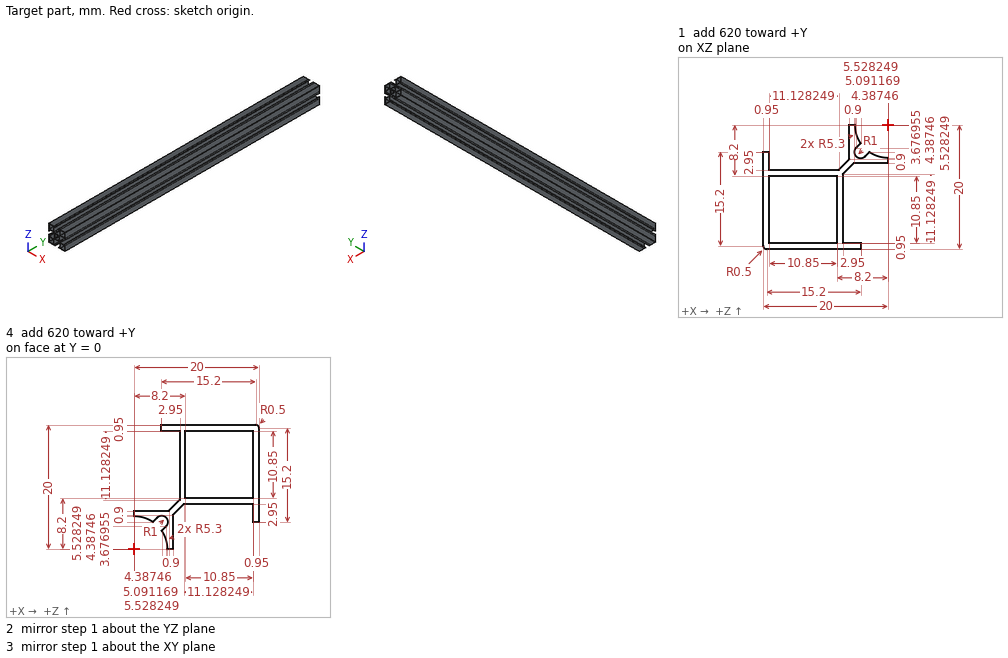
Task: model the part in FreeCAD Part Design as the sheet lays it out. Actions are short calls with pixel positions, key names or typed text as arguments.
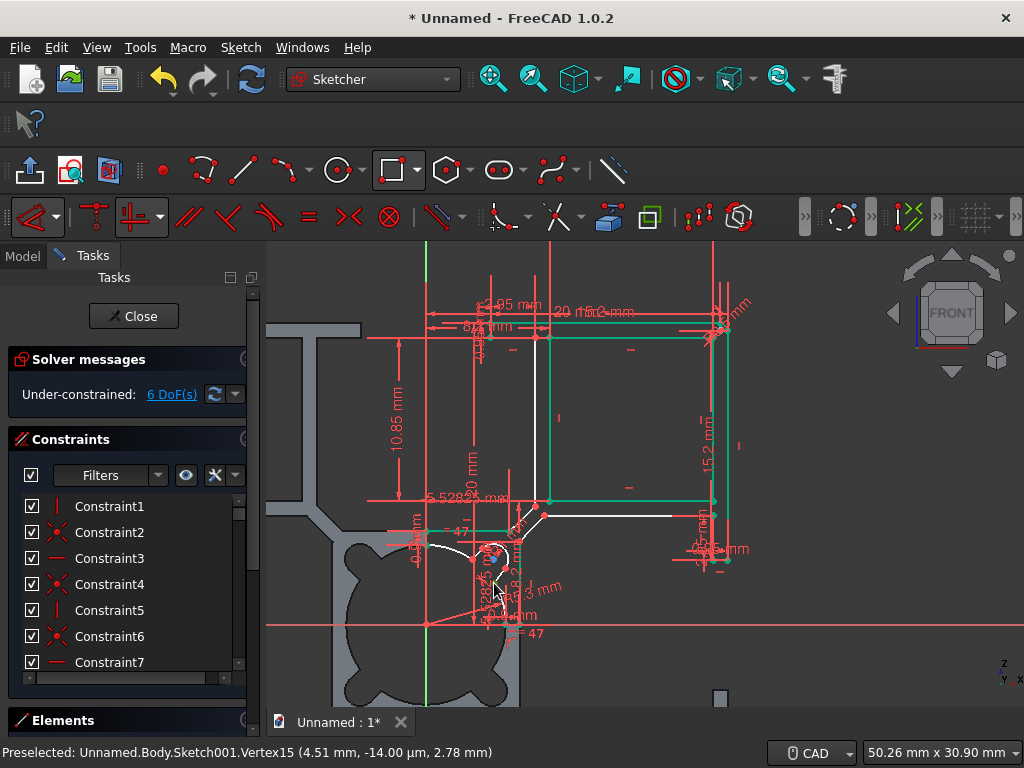
click(58, 218)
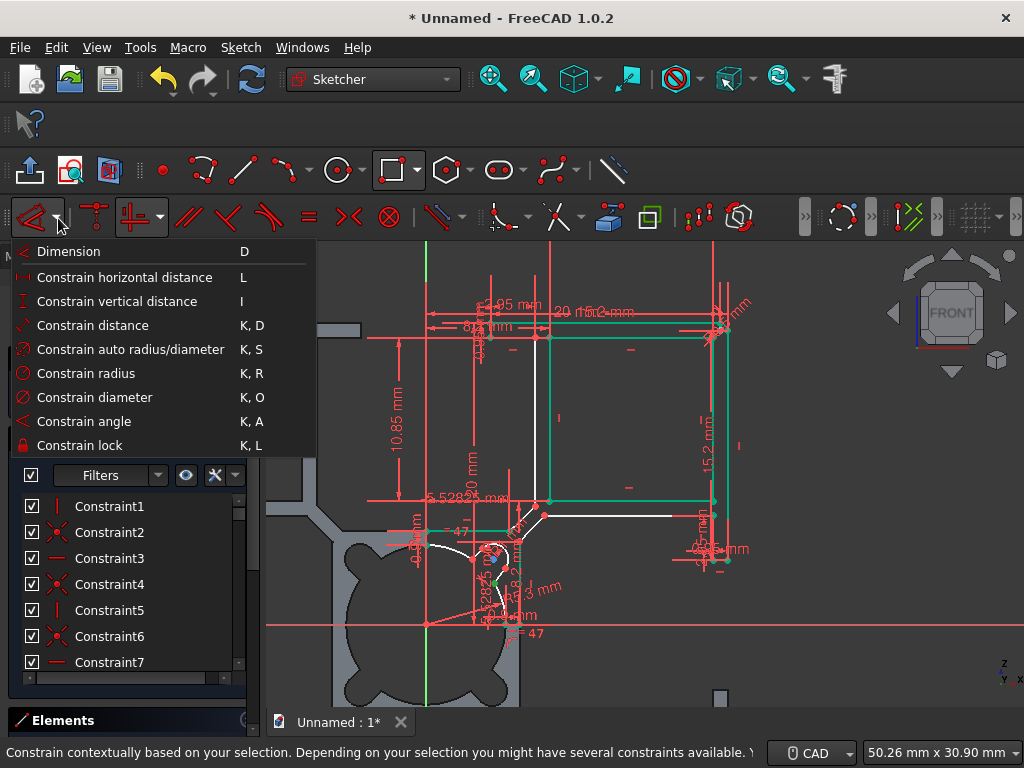
click(164, 277)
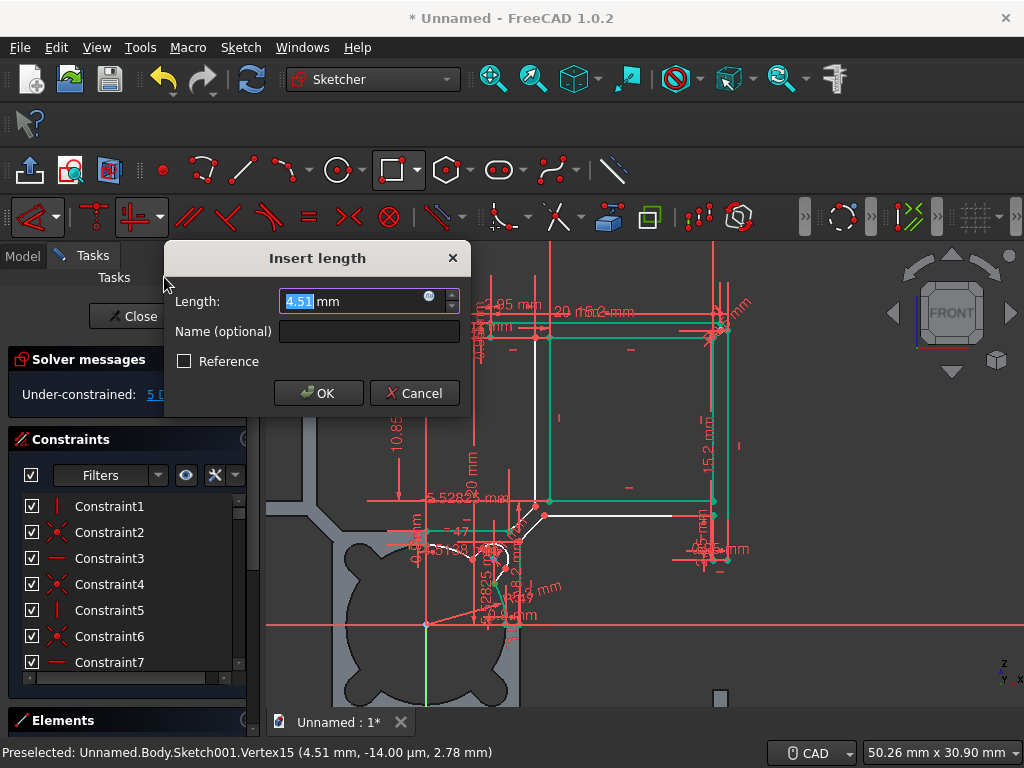
text(4.38746)
key(Return)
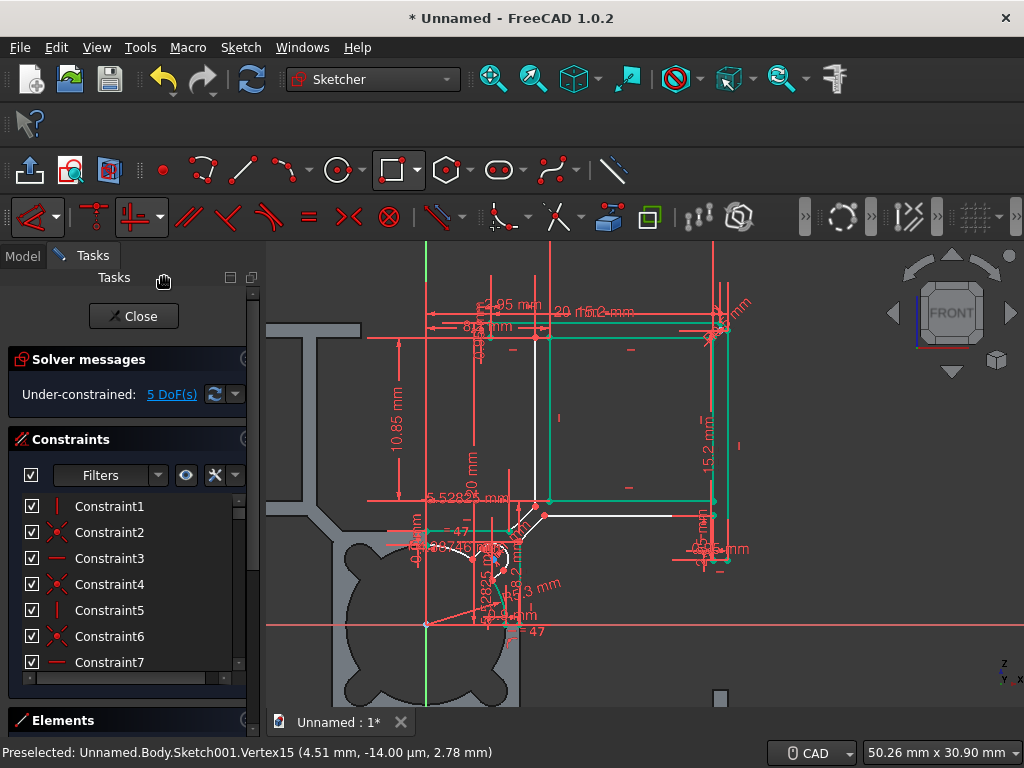
click(472, 560)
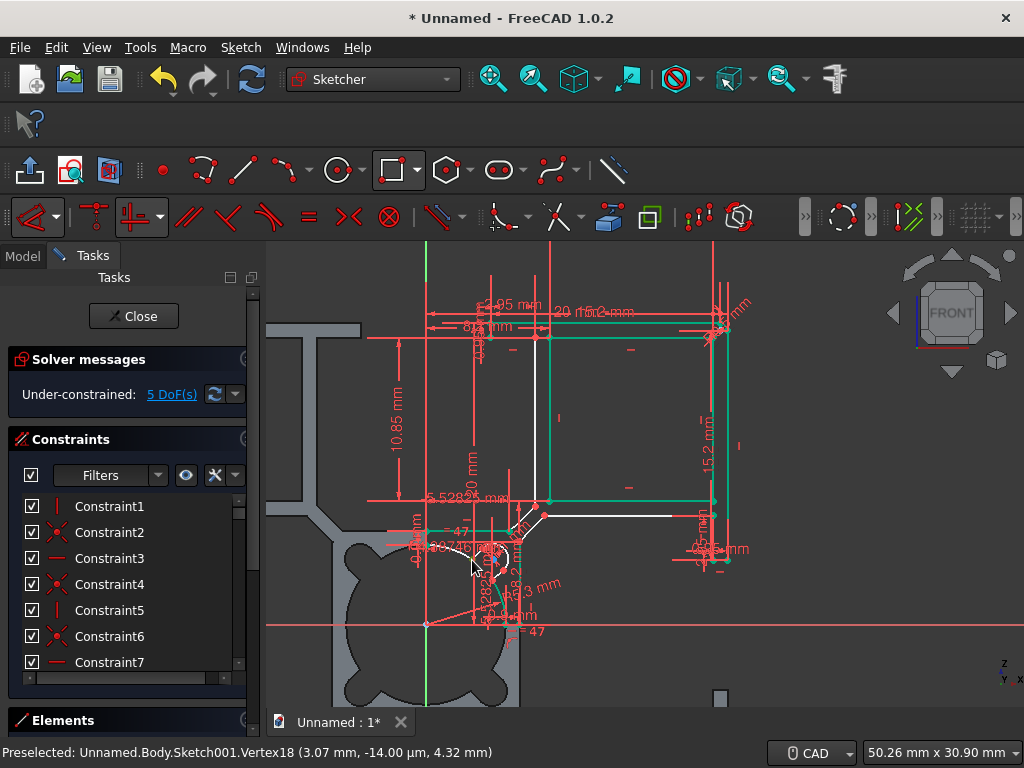
key(i)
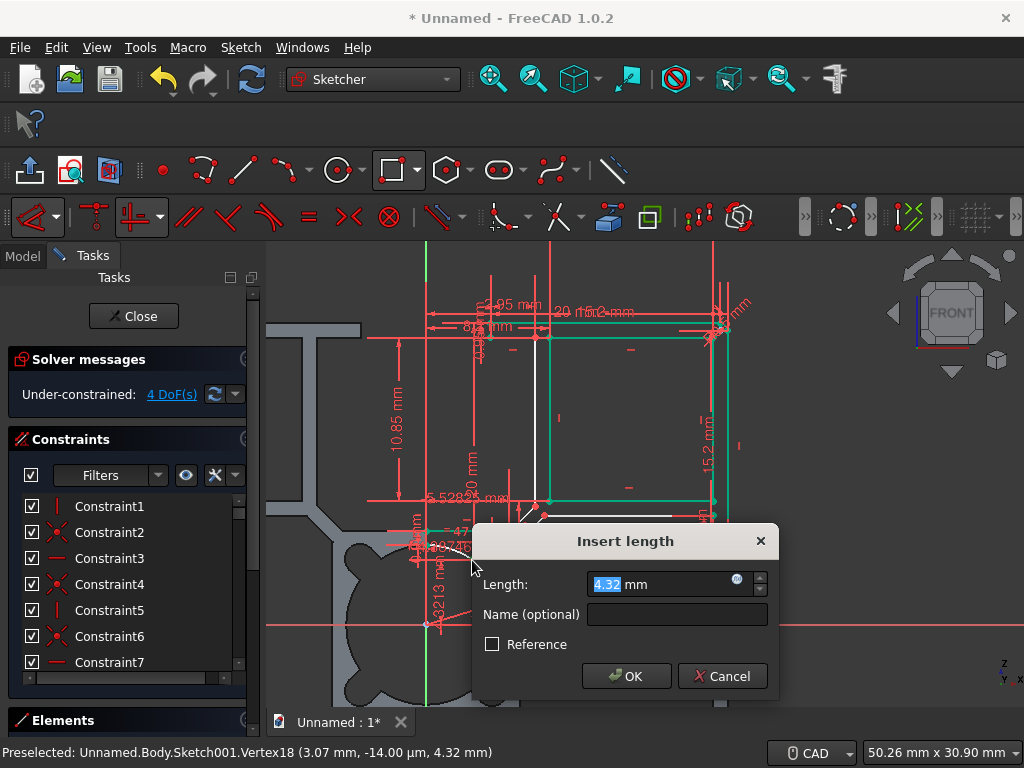
text(4.38746)
key(Return)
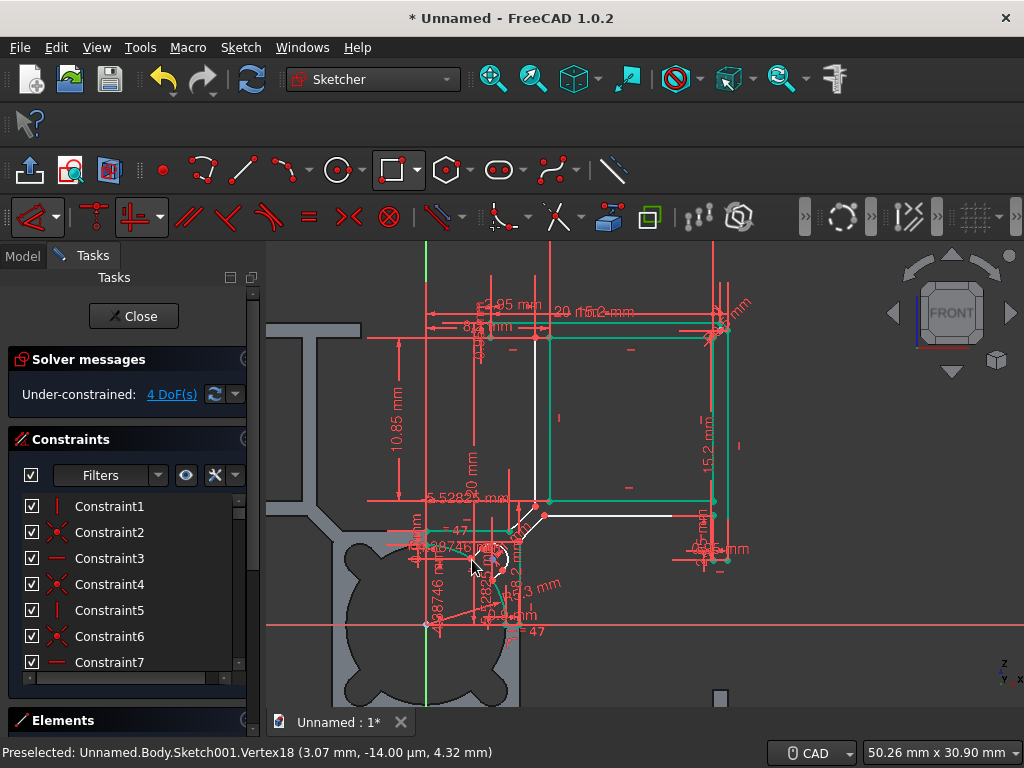
click(663, 516)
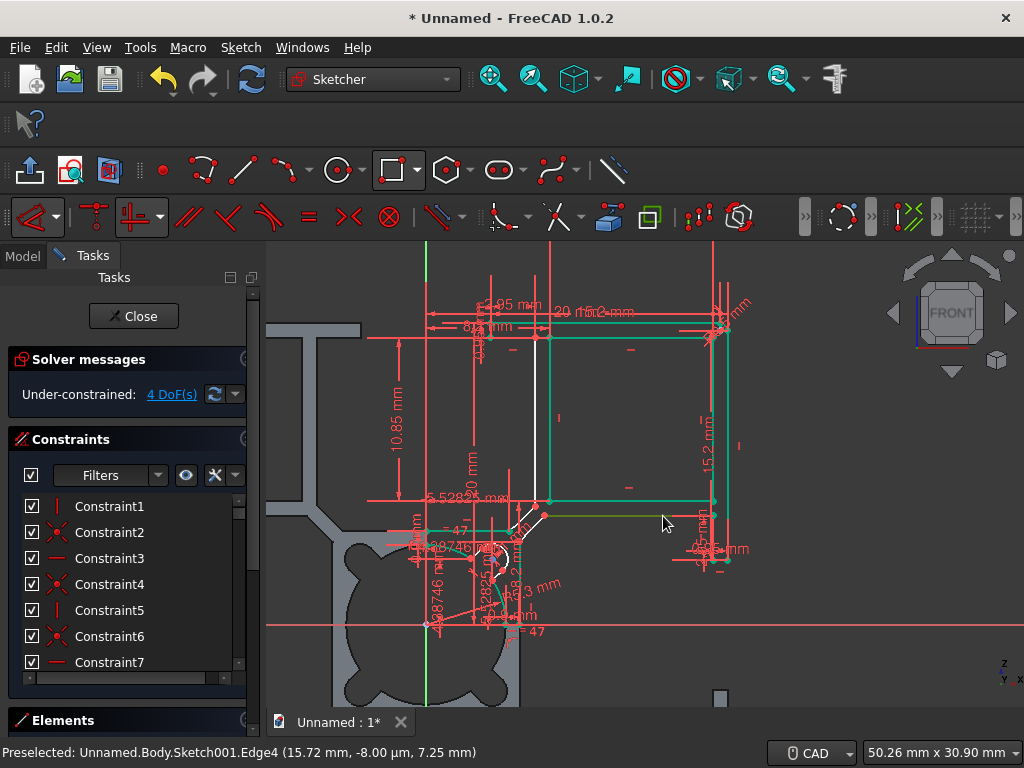
click(58, 218)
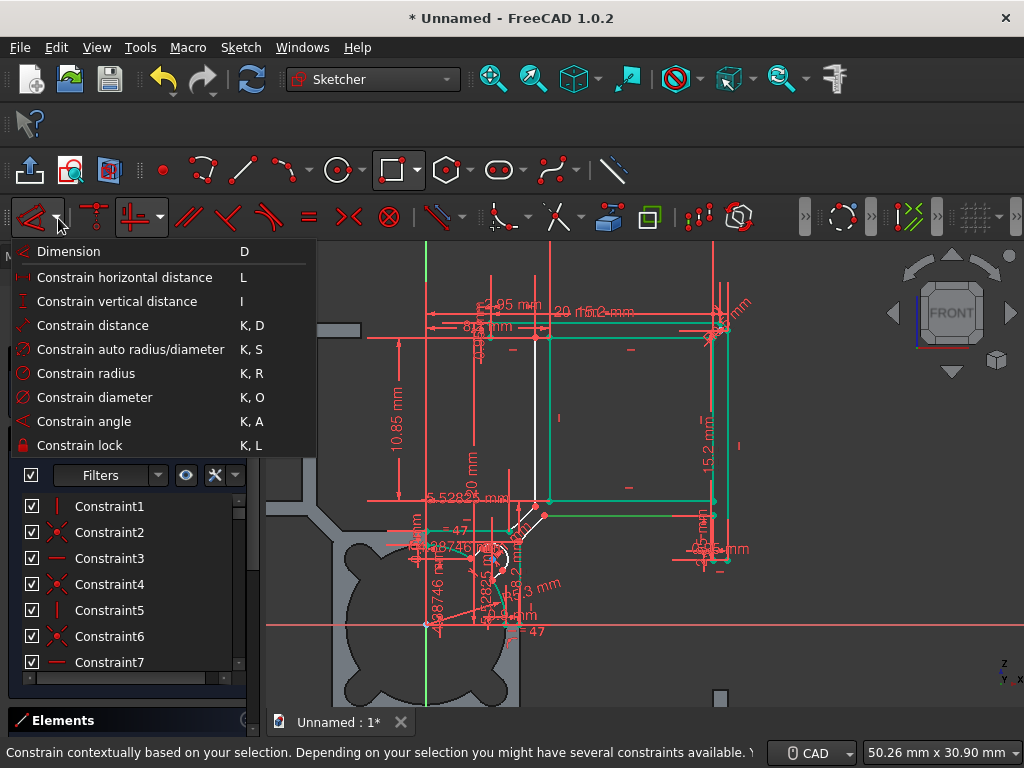
click(164, 277)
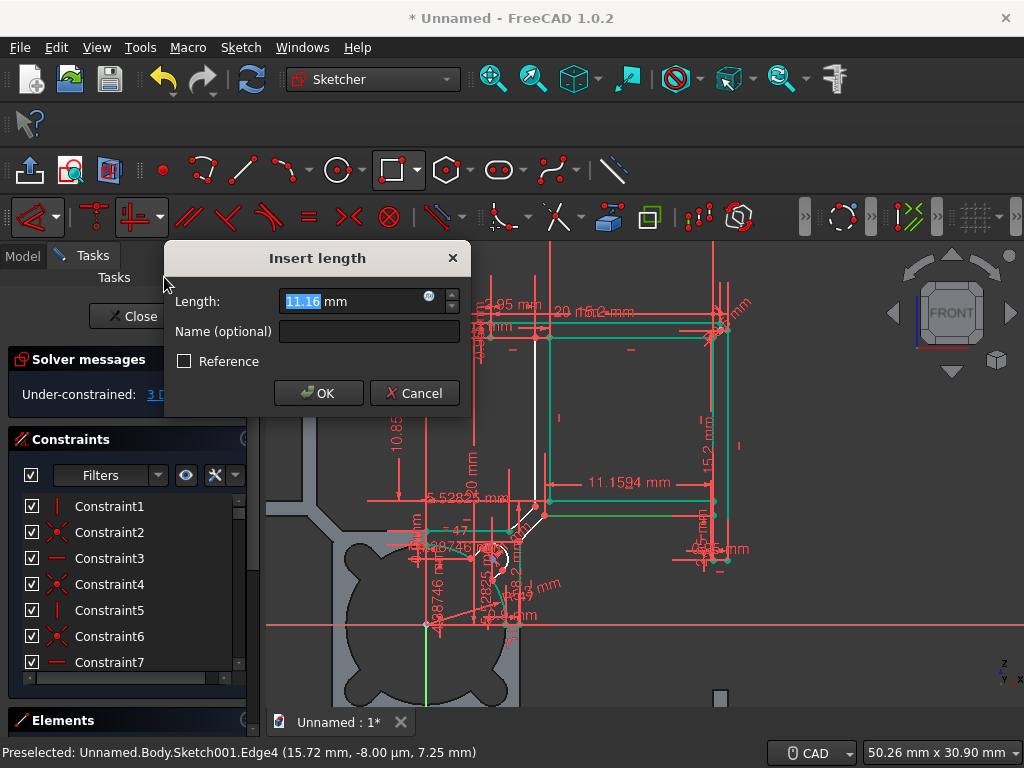
text(11.128249)
key(Return)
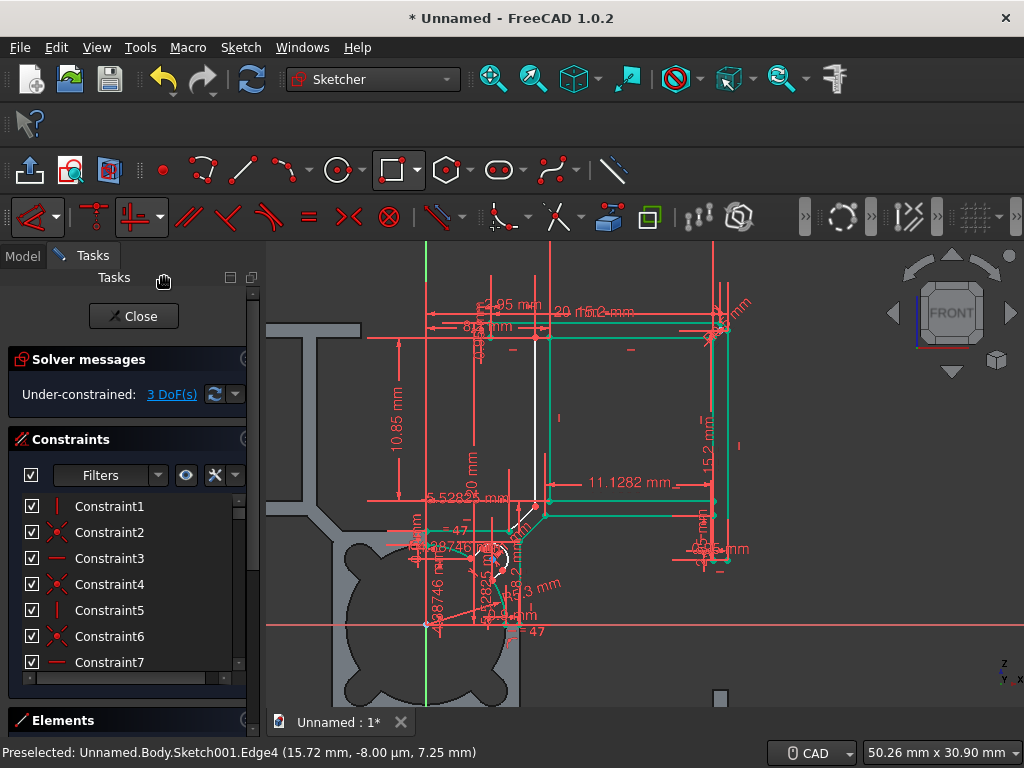
click(535, 456)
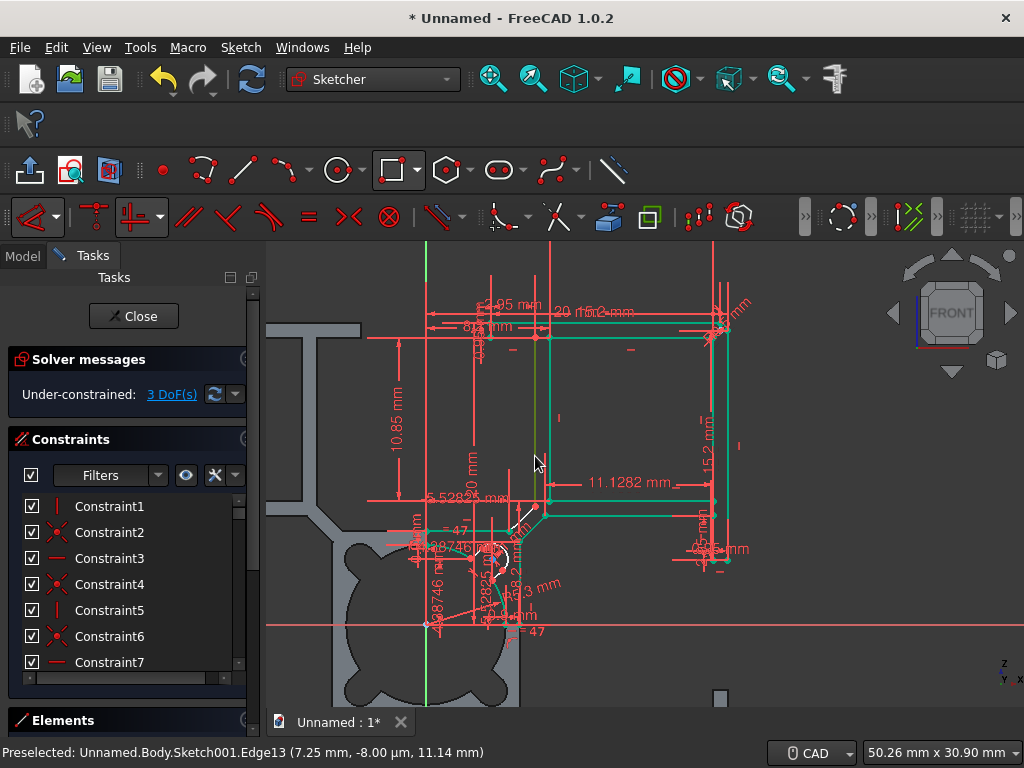
click(58, 218)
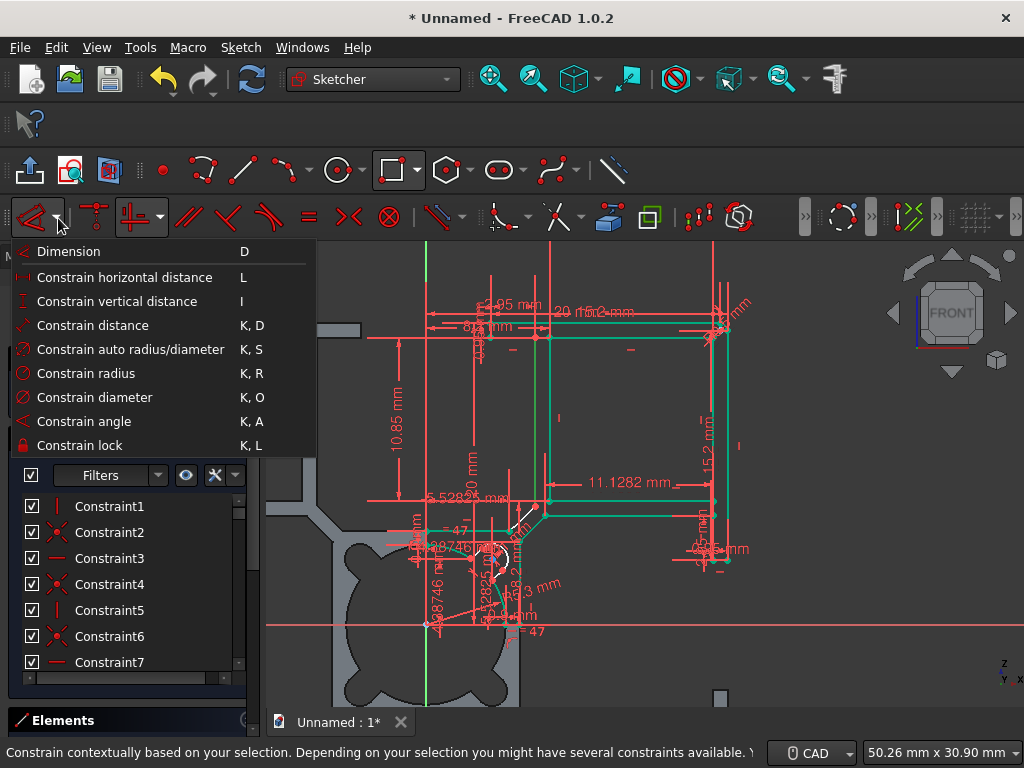
click(164, 301)